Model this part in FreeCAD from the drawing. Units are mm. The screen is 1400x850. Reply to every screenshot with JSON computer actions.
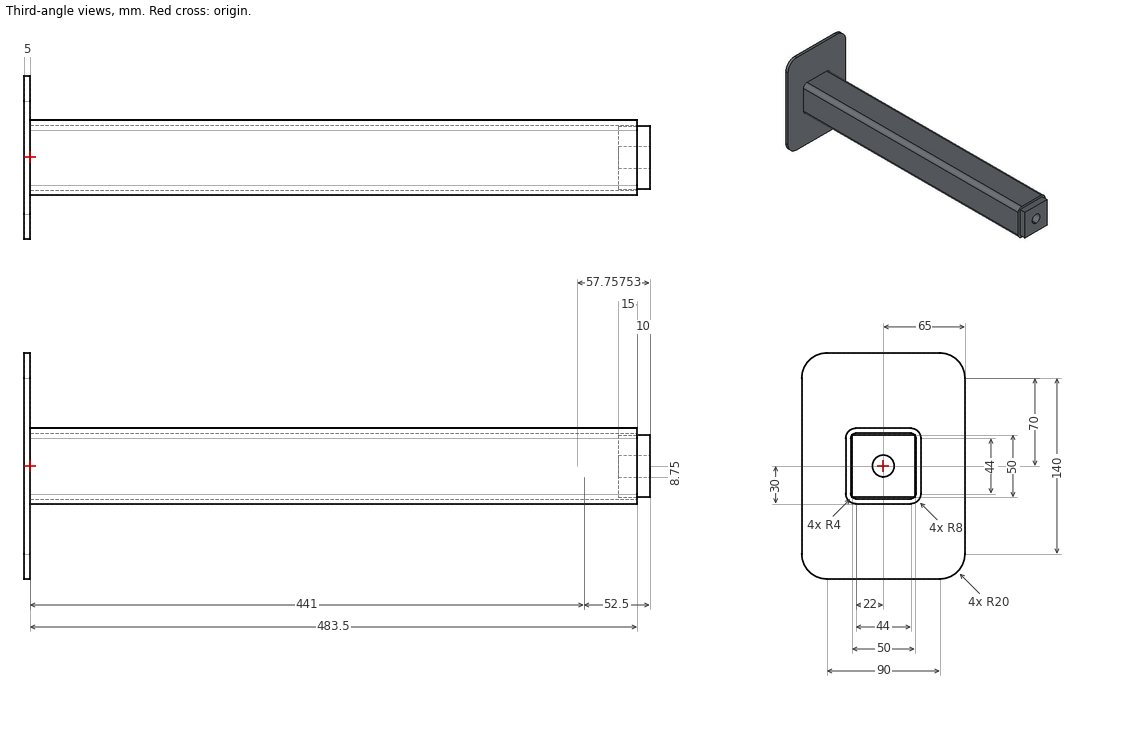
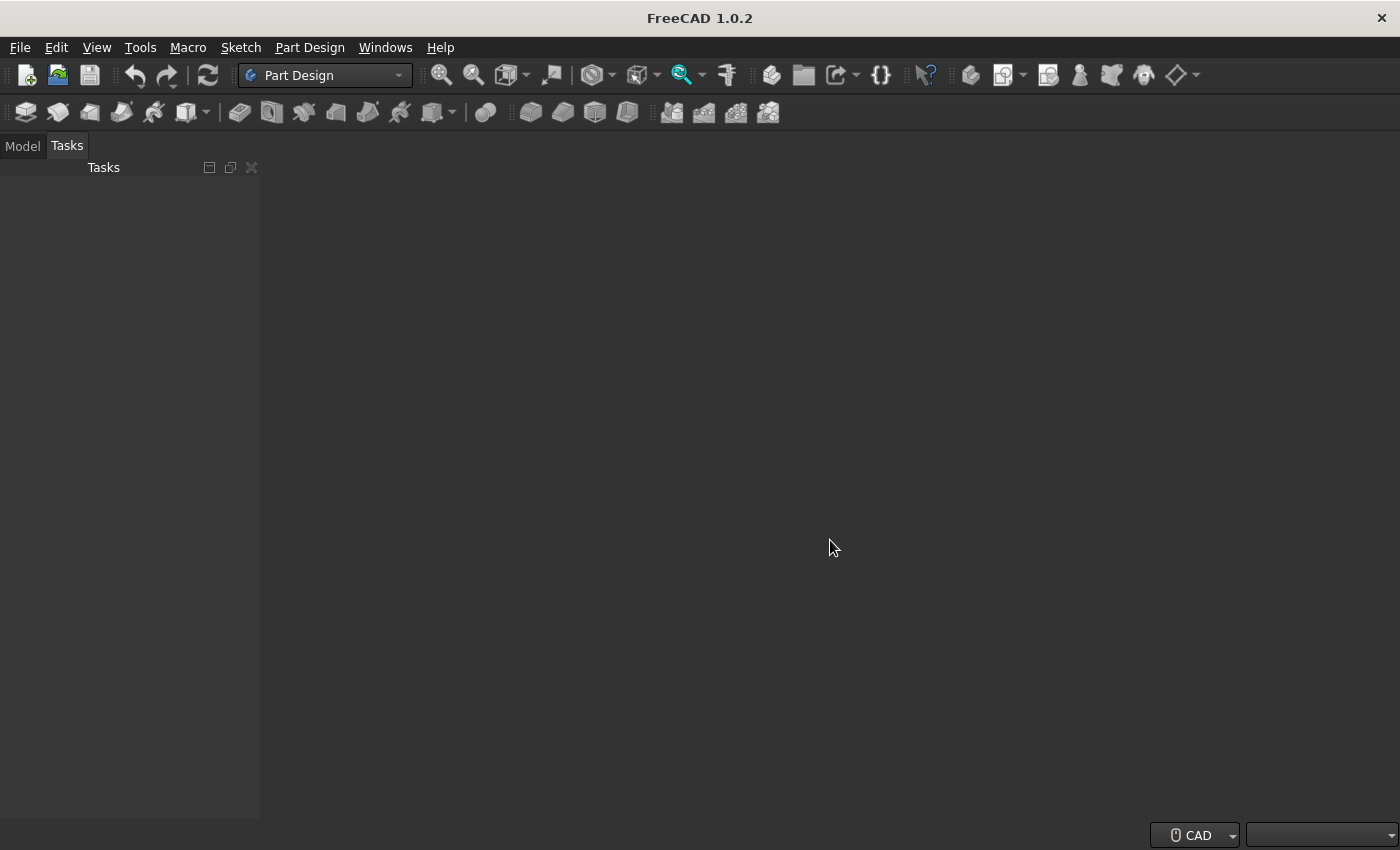
{"action": "left_click", "coordinate": [26, 76]}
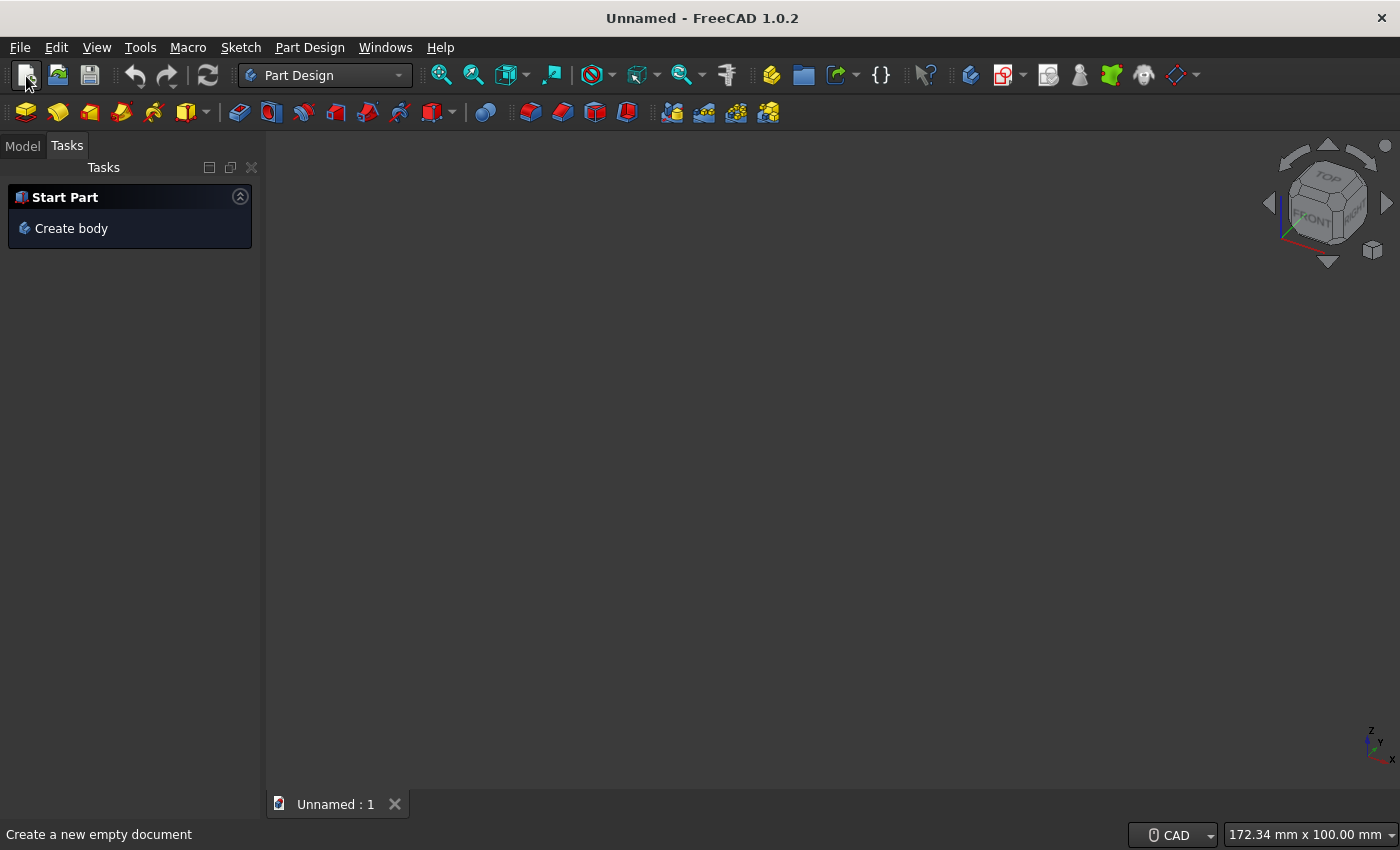
{"action": "left_click", "coordinate": [1004, 76]}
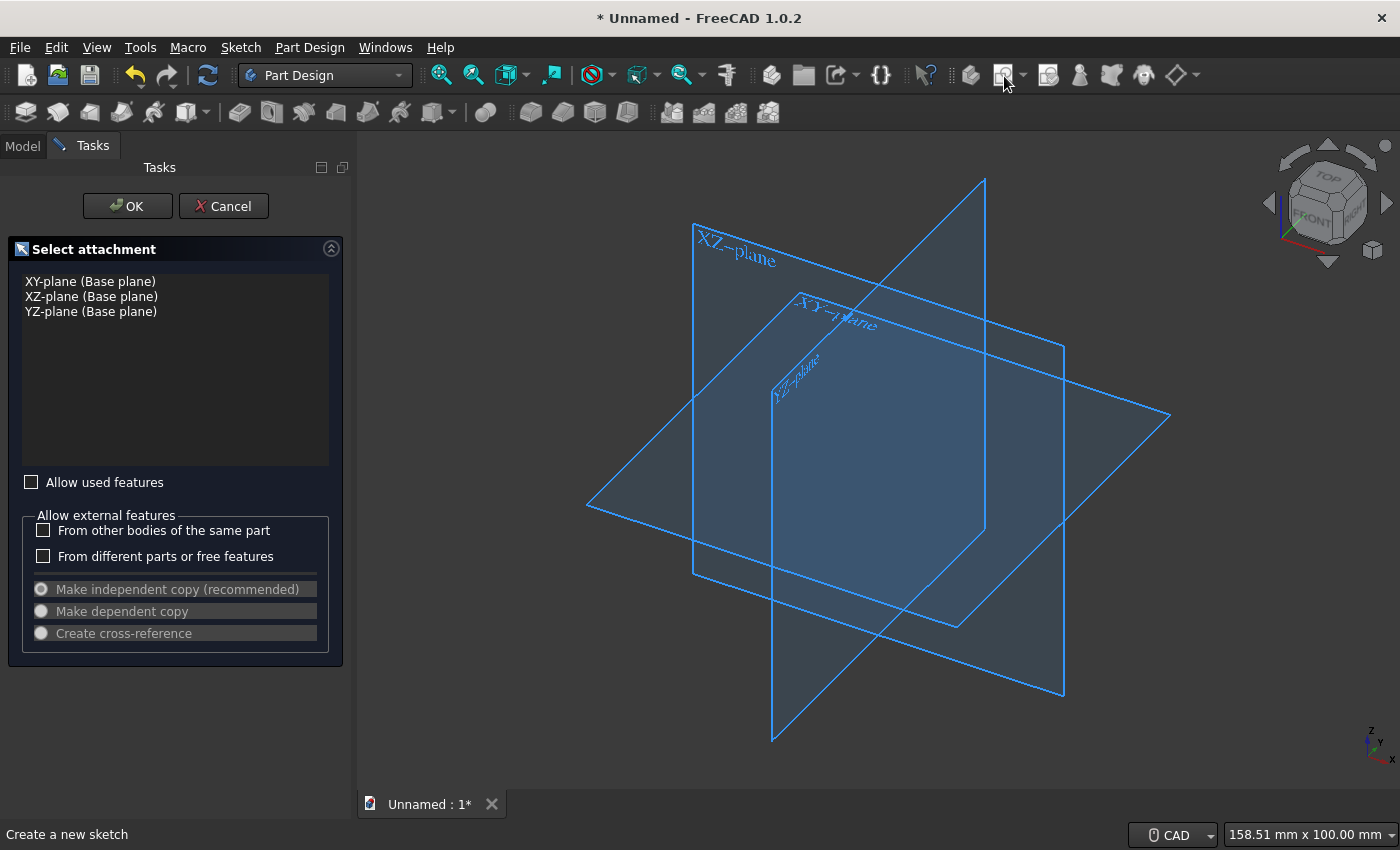
{"action": "left_click", "coordinate": [82, 312]}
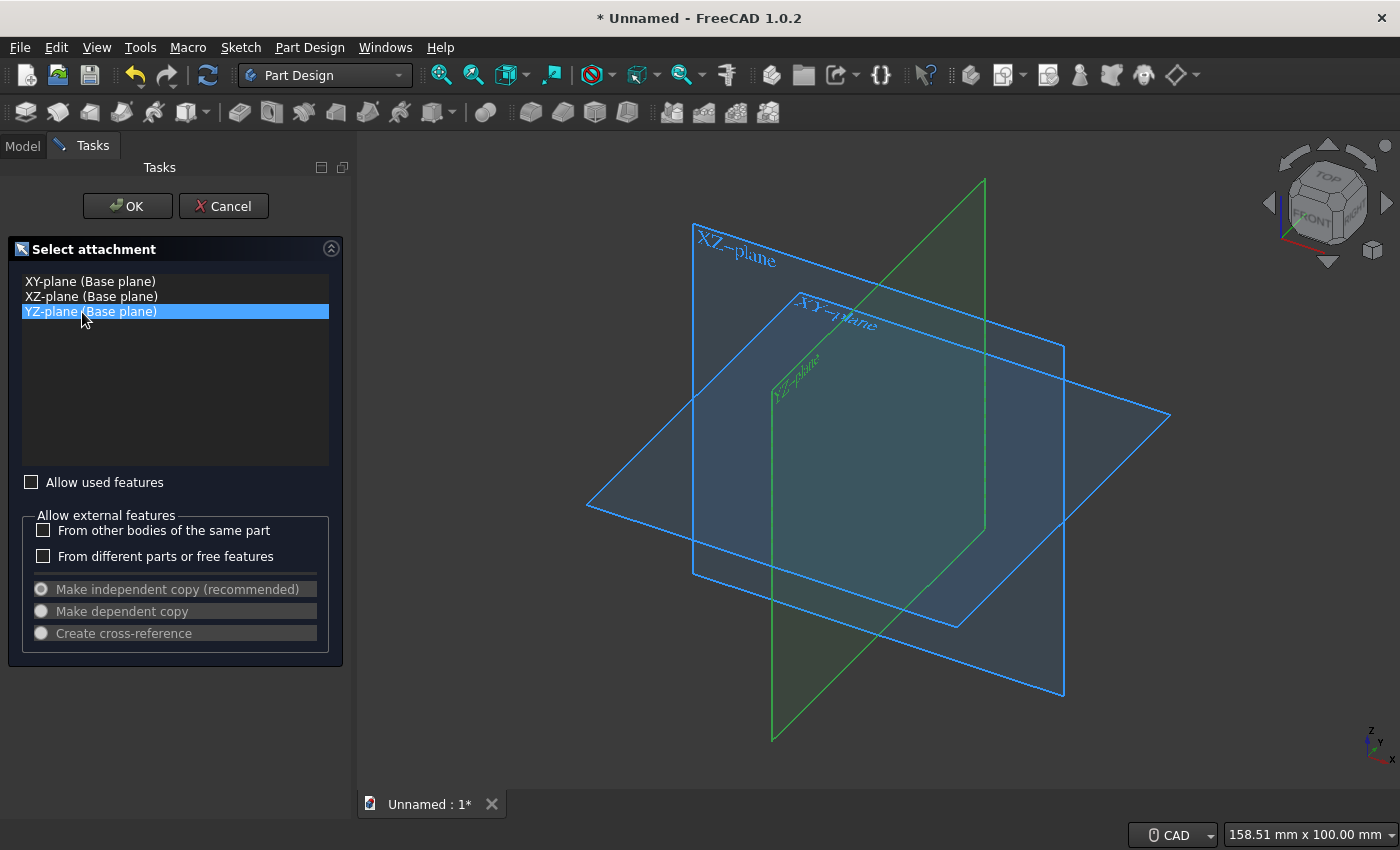
{"action": "left_click", "coordinate": [128, 206]}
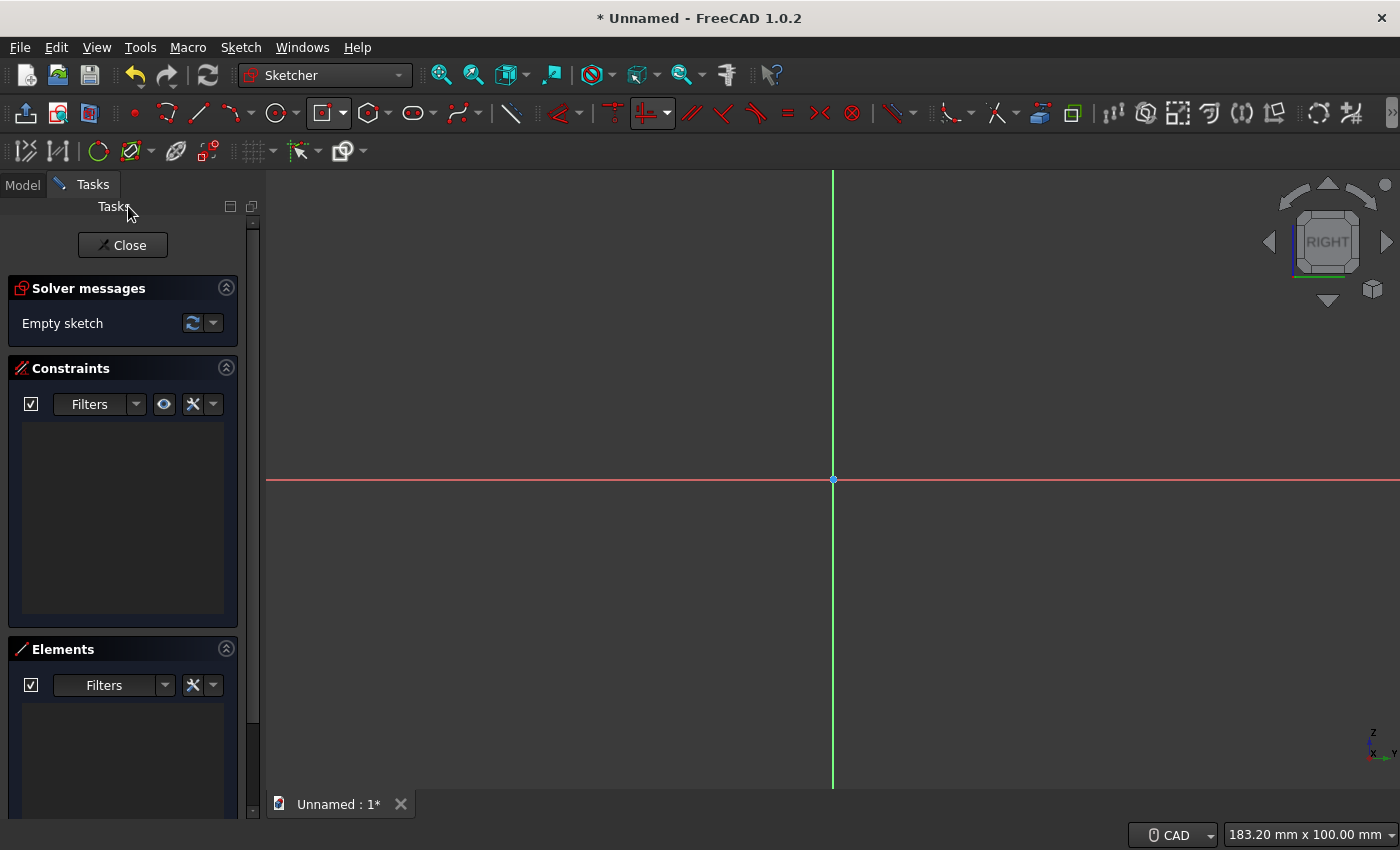
{"action": "left_click", "coordinate": [200, 114]}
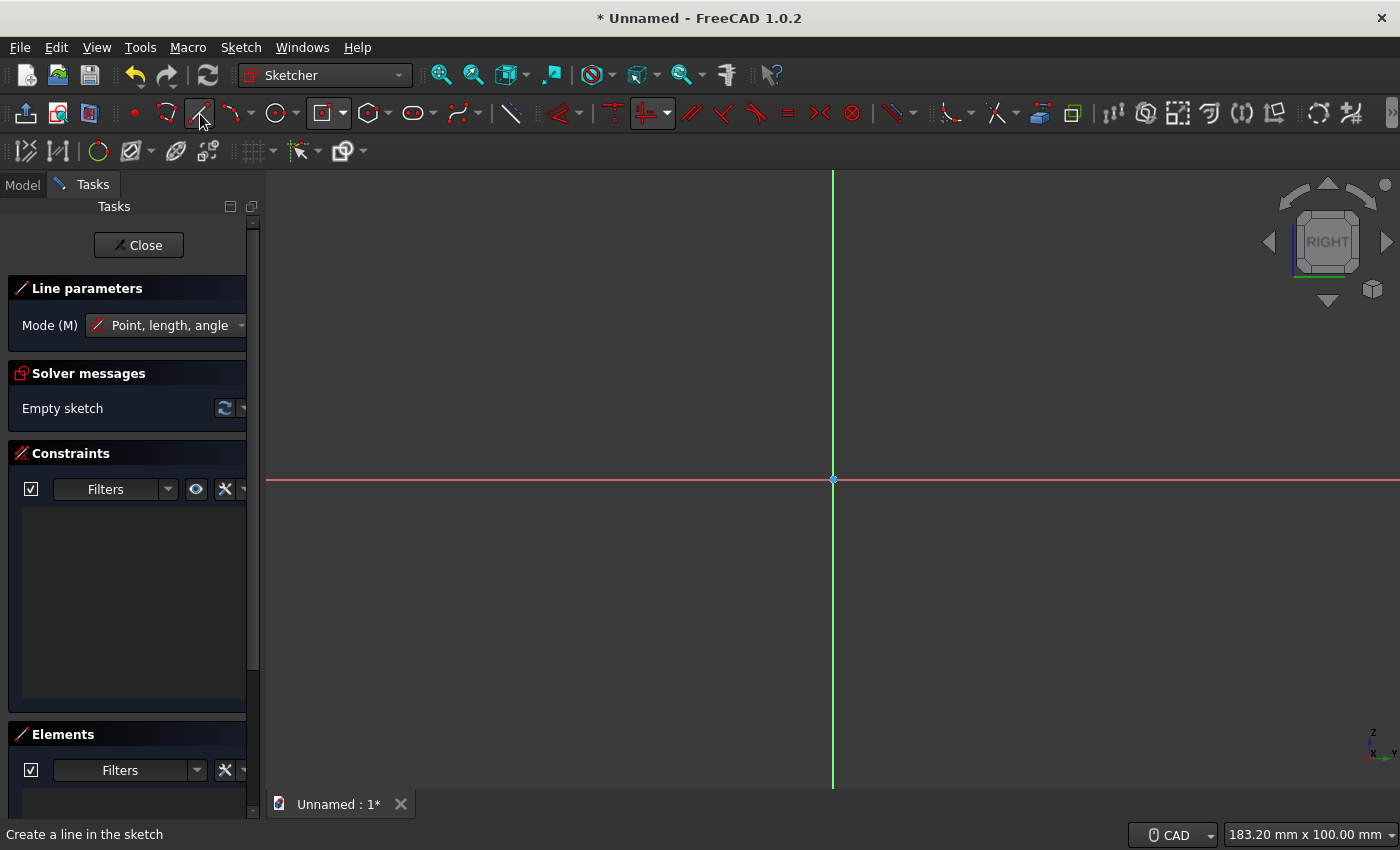
{"action": "left_click", "coordinate": [697, 665]}
{"action": "left_click", "coordinate": [969, 665]}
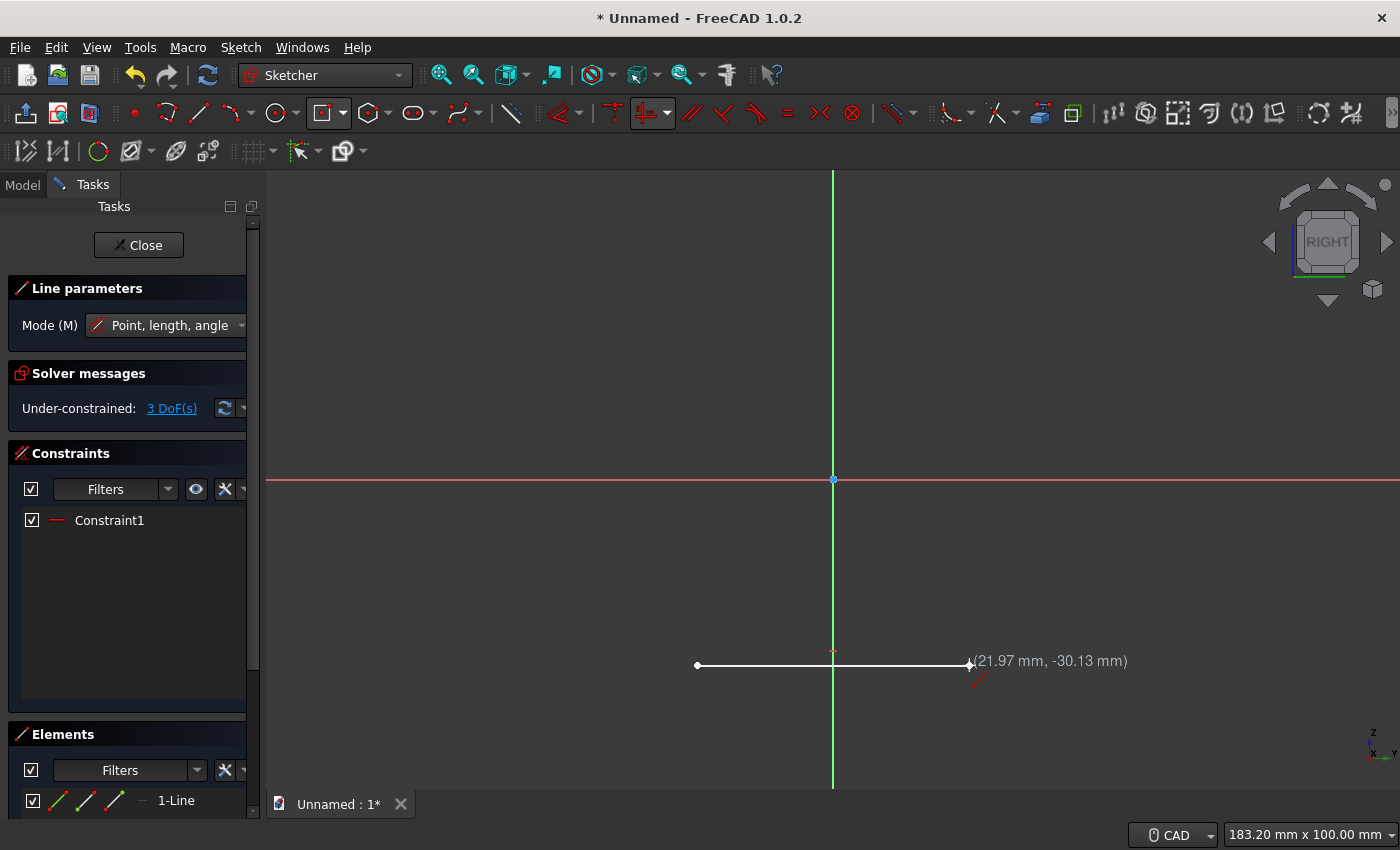
{"action": "left_click", "coordinate": [1019, 616]}
{"action": "left_click", "coordinate": [1019, 343]}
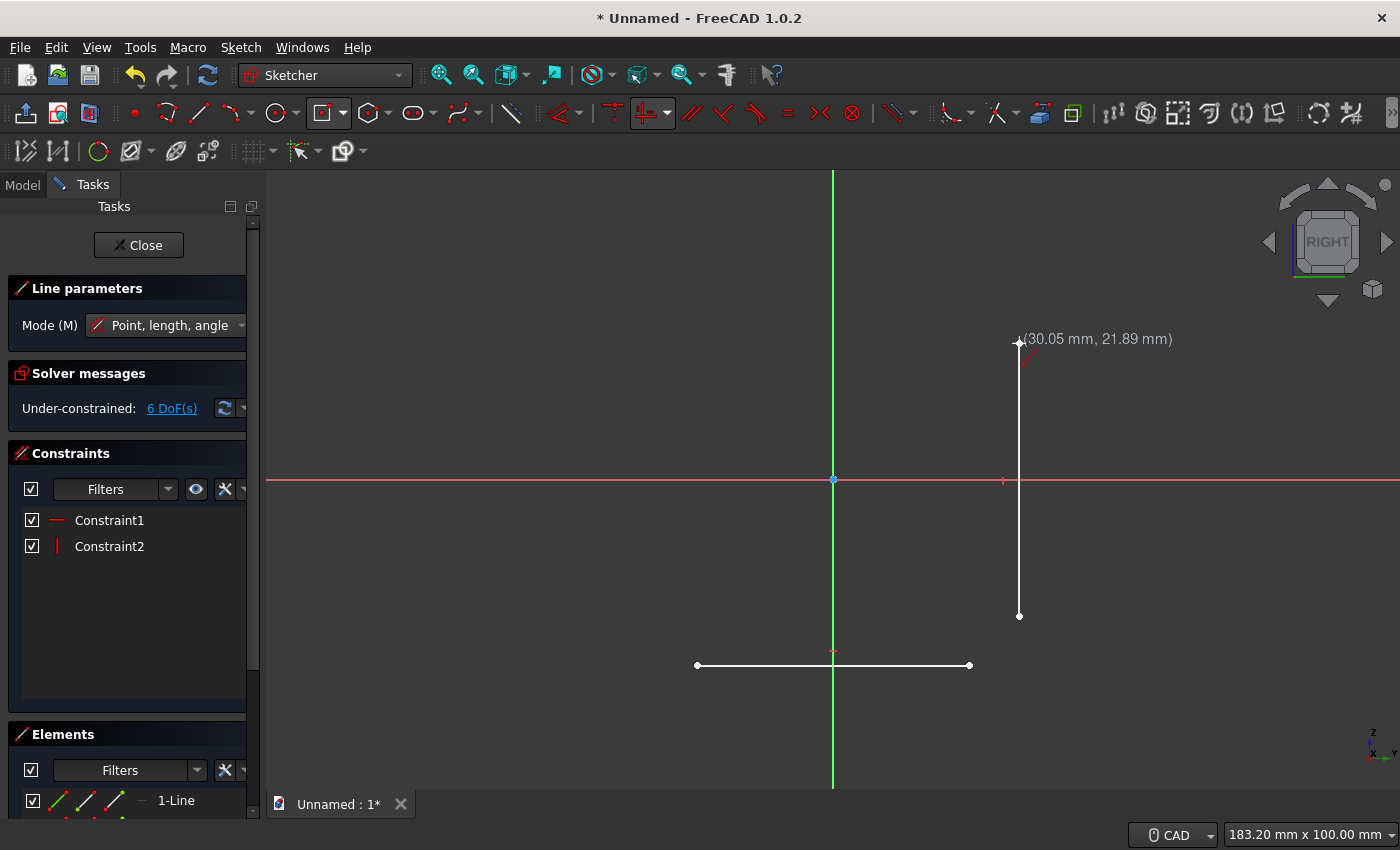
{"action": "left_click", "coordinate": [969, 294]}
{"action": "left_click", "coordinate": [697, 294]}